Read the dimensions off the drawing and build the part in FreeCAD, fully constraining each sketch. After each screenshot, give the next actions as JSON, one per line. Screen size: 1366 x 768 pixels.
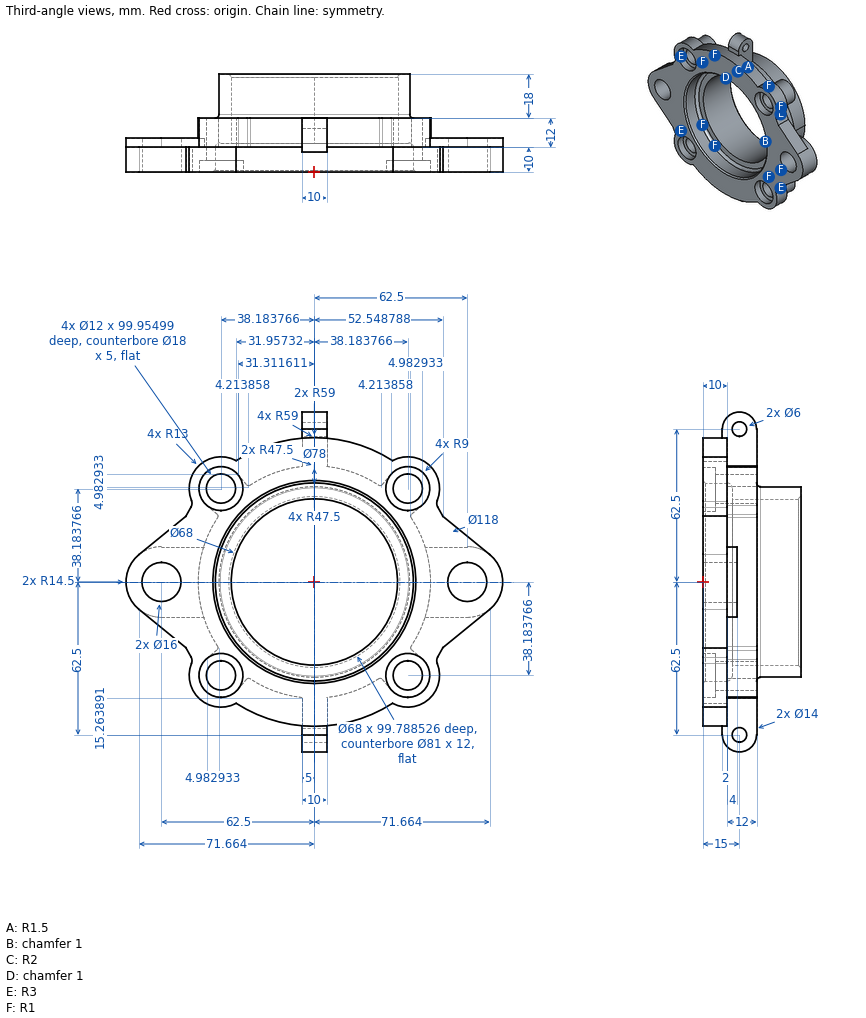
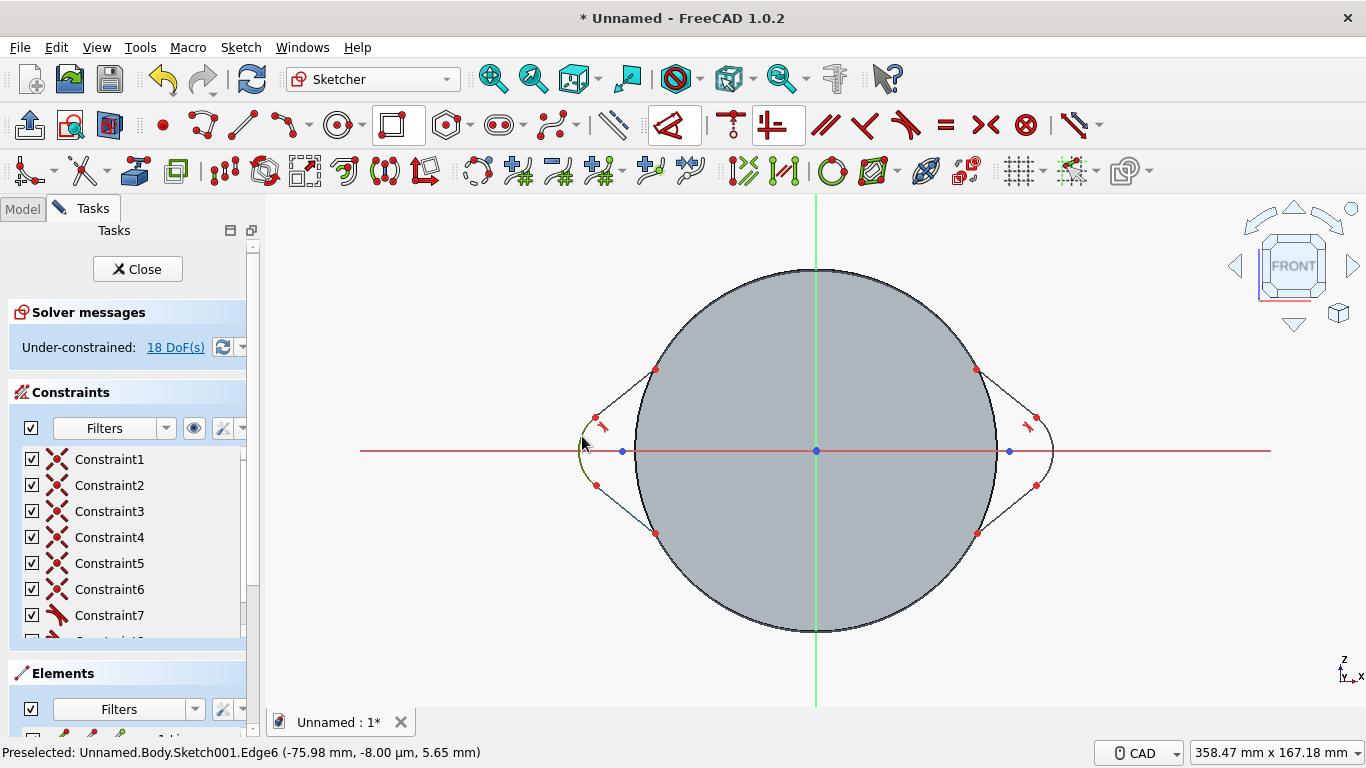
{"action": "left_click", "coordinate": [906, 126]}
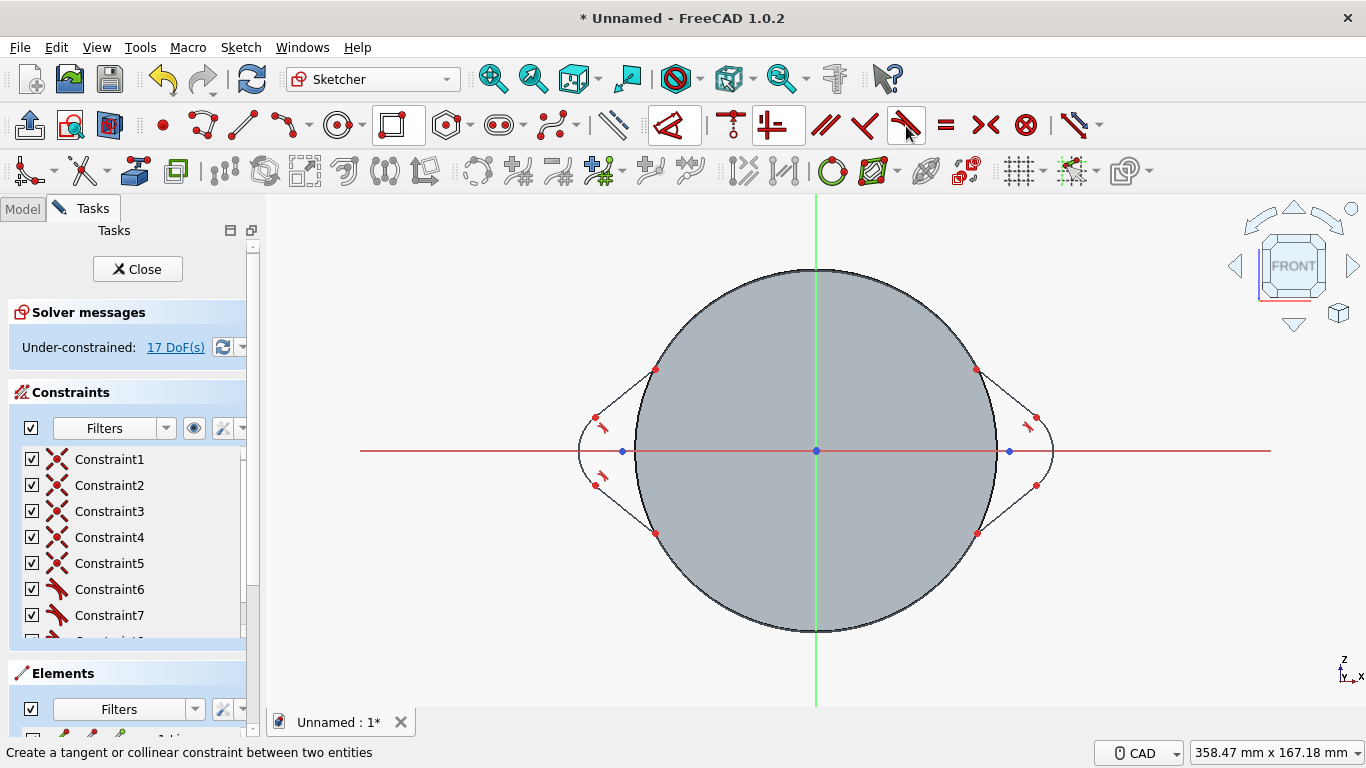
{"action": "left_click", "coordinate": [995, 520]}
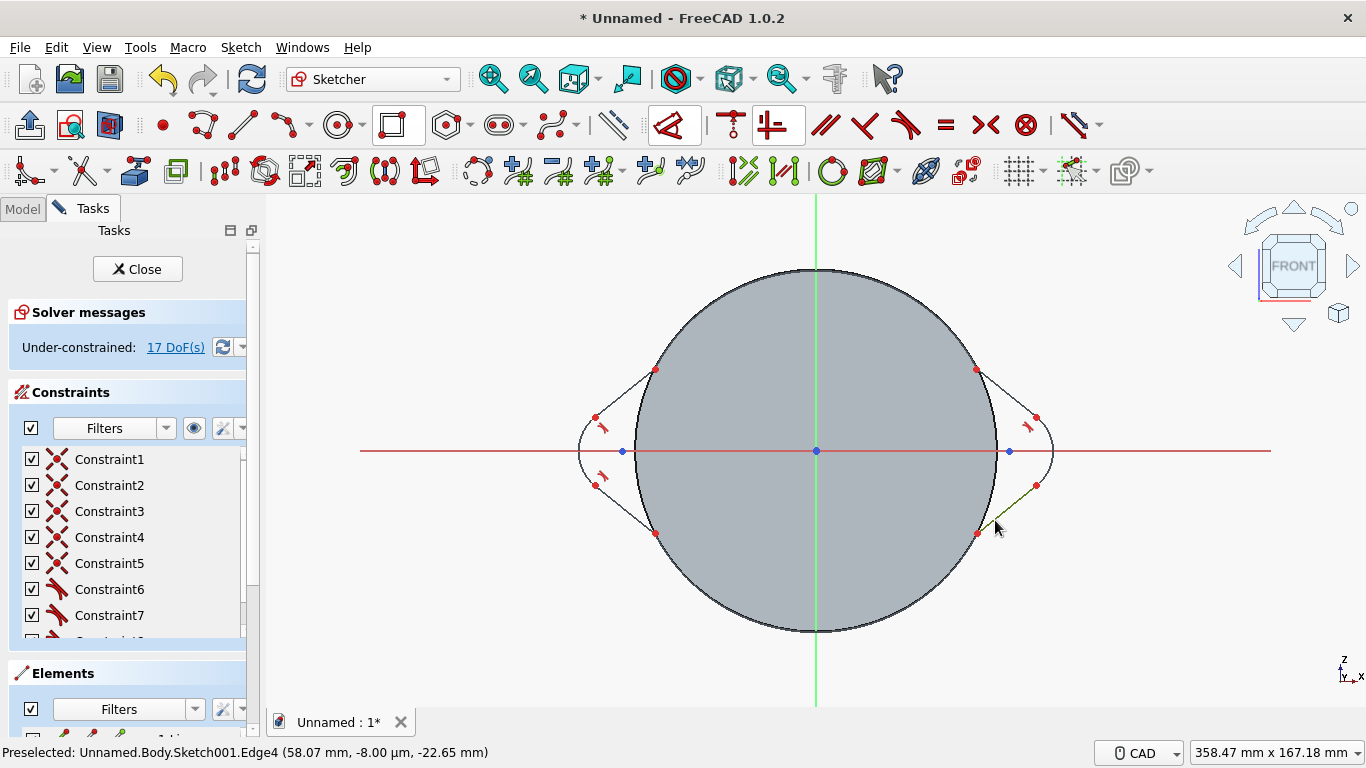
{"action": "left_click", "coordinate": [1050, 467]}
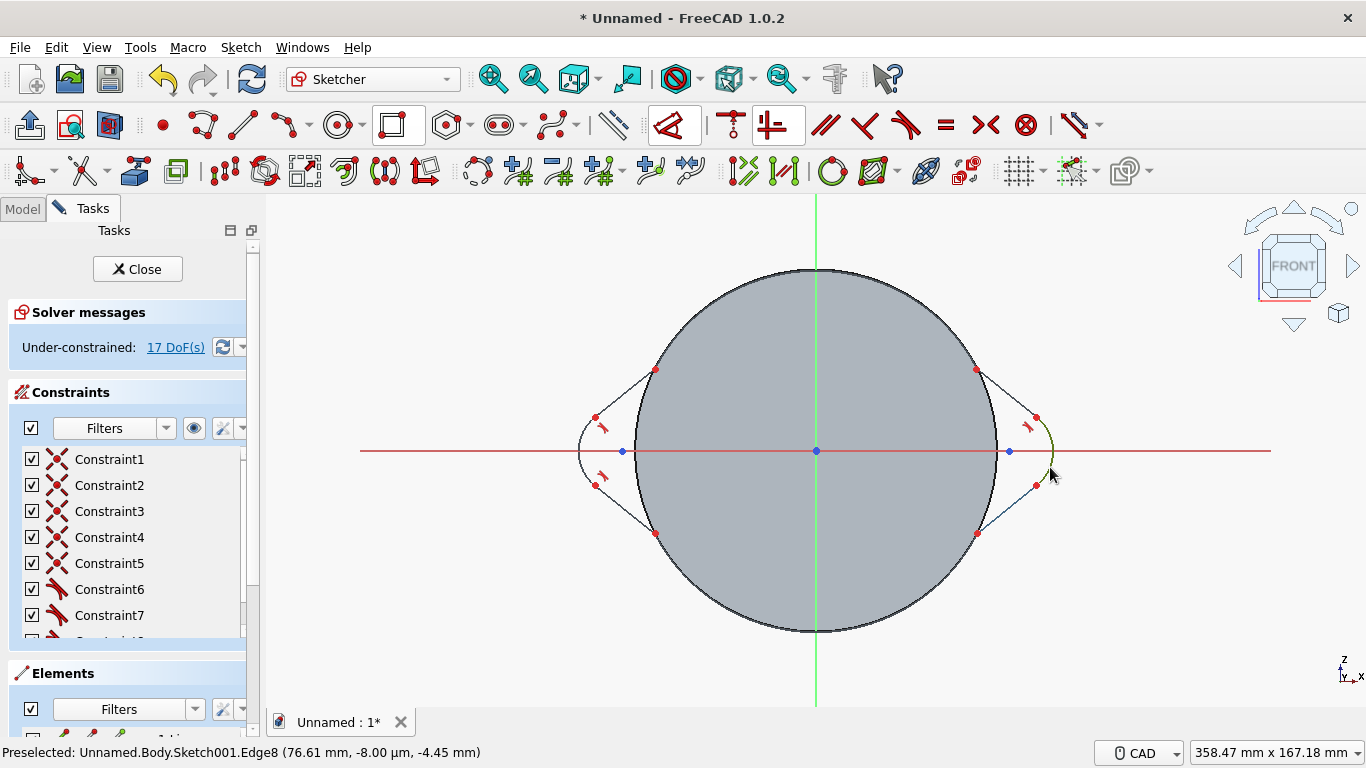
{"action": "left_click", "coordinate": [906, 126]}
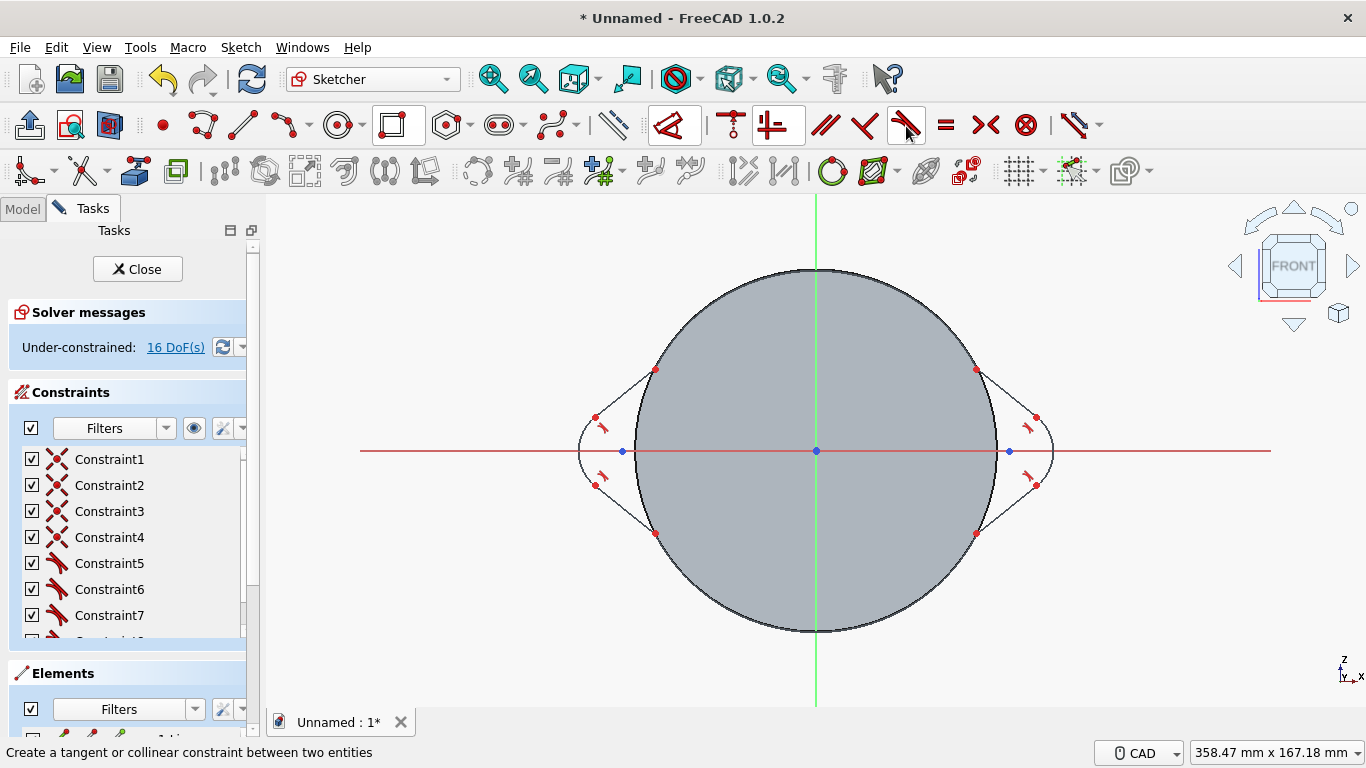
{"action": "left_click", "coordinate": [893, 288]}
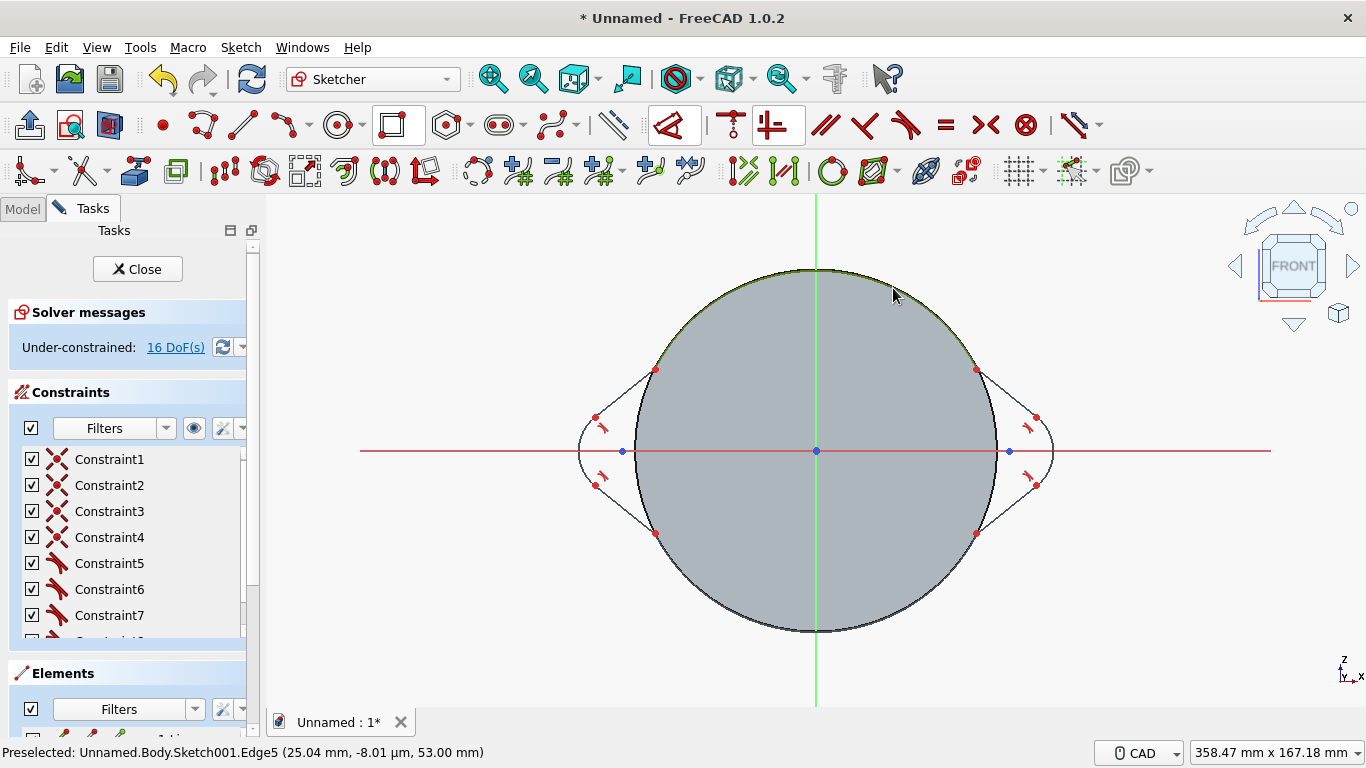
{"action": "left_click", "coordinate": [739, 615]}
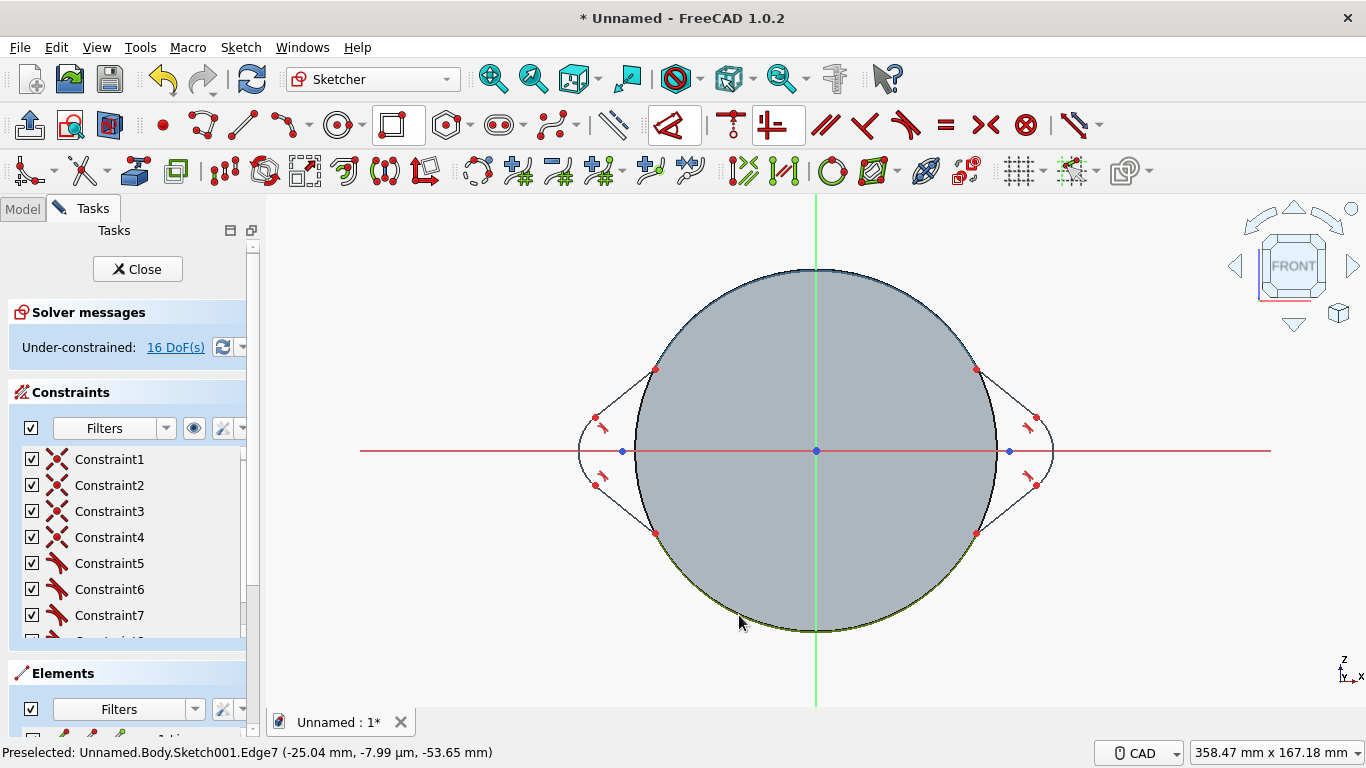
{"action": "left_click", "coordinate": [732, 126]}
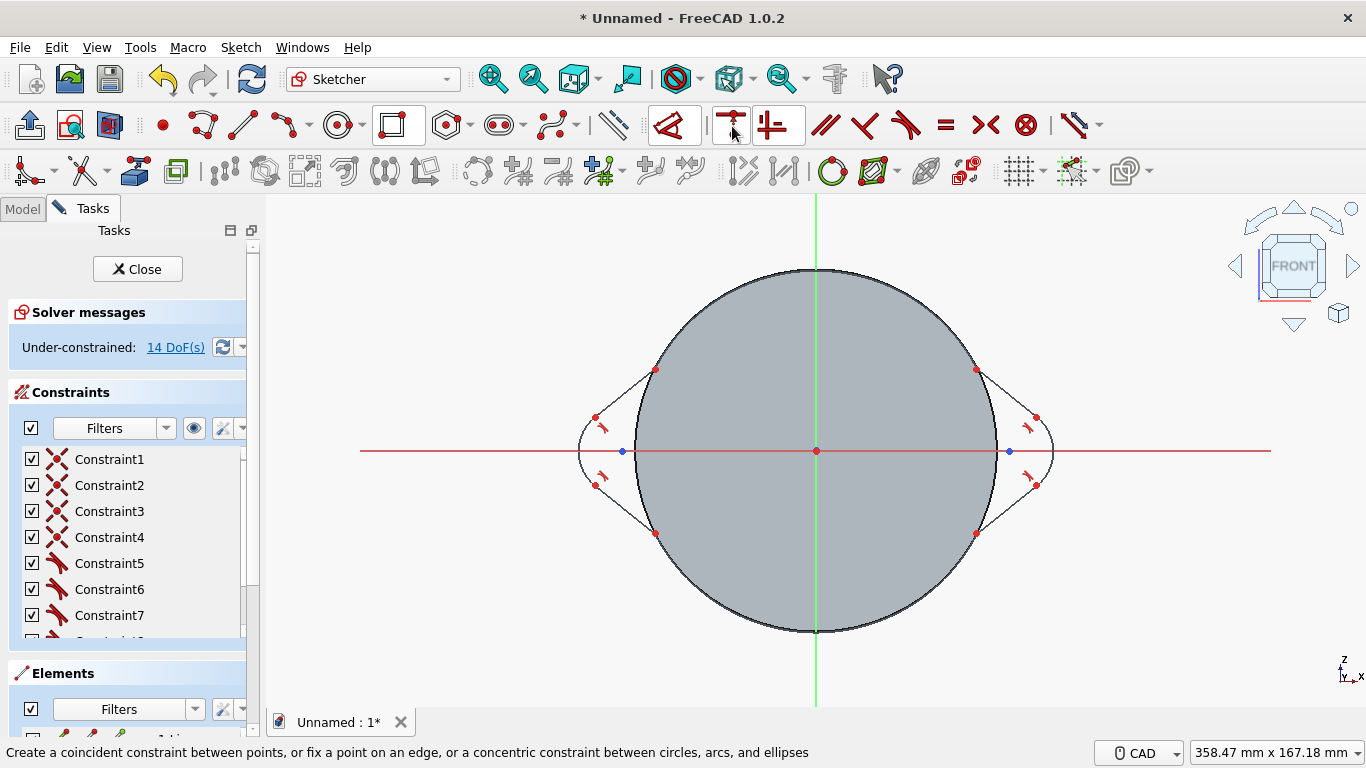
{"action": "left_click_drag", "start_coordinate": [806, 440], "coordinate": [826, 462]}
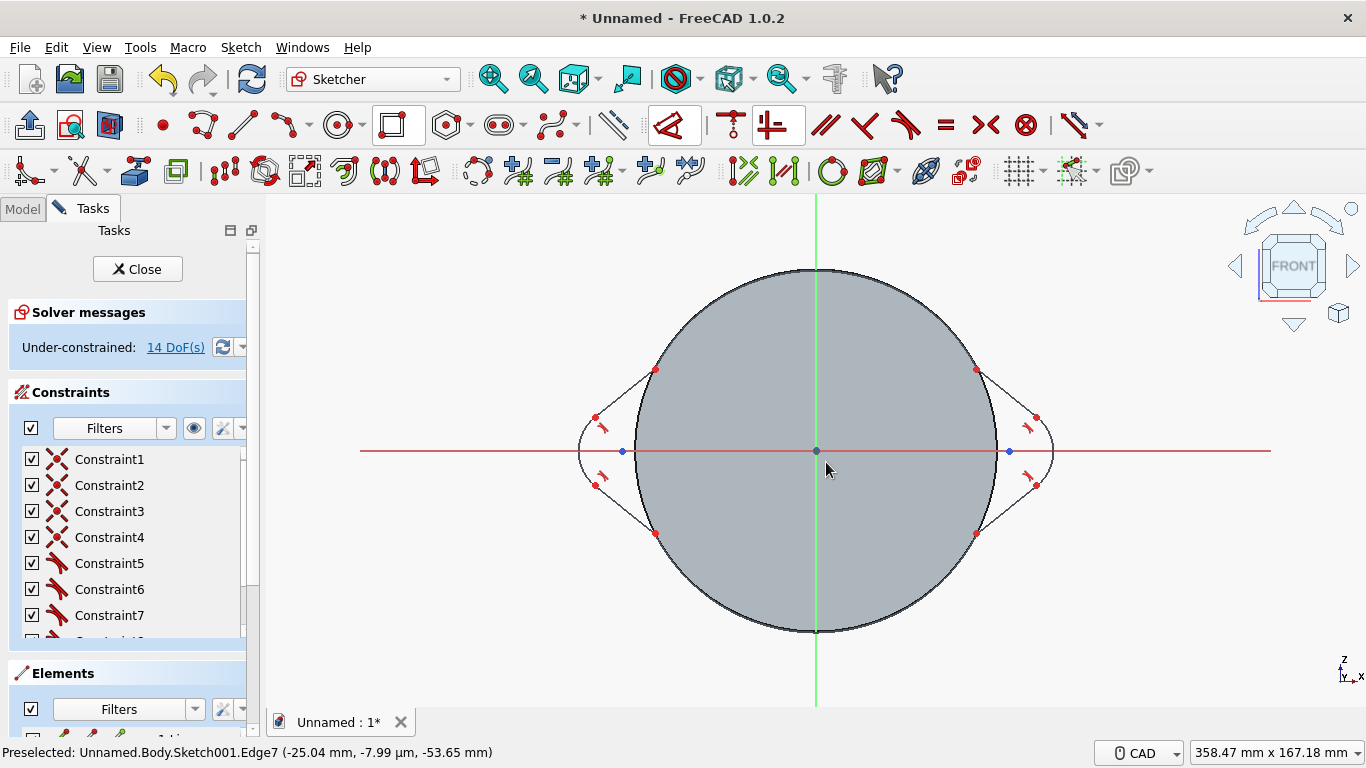
{"action": "left_click", "coordinate": [732, 126]}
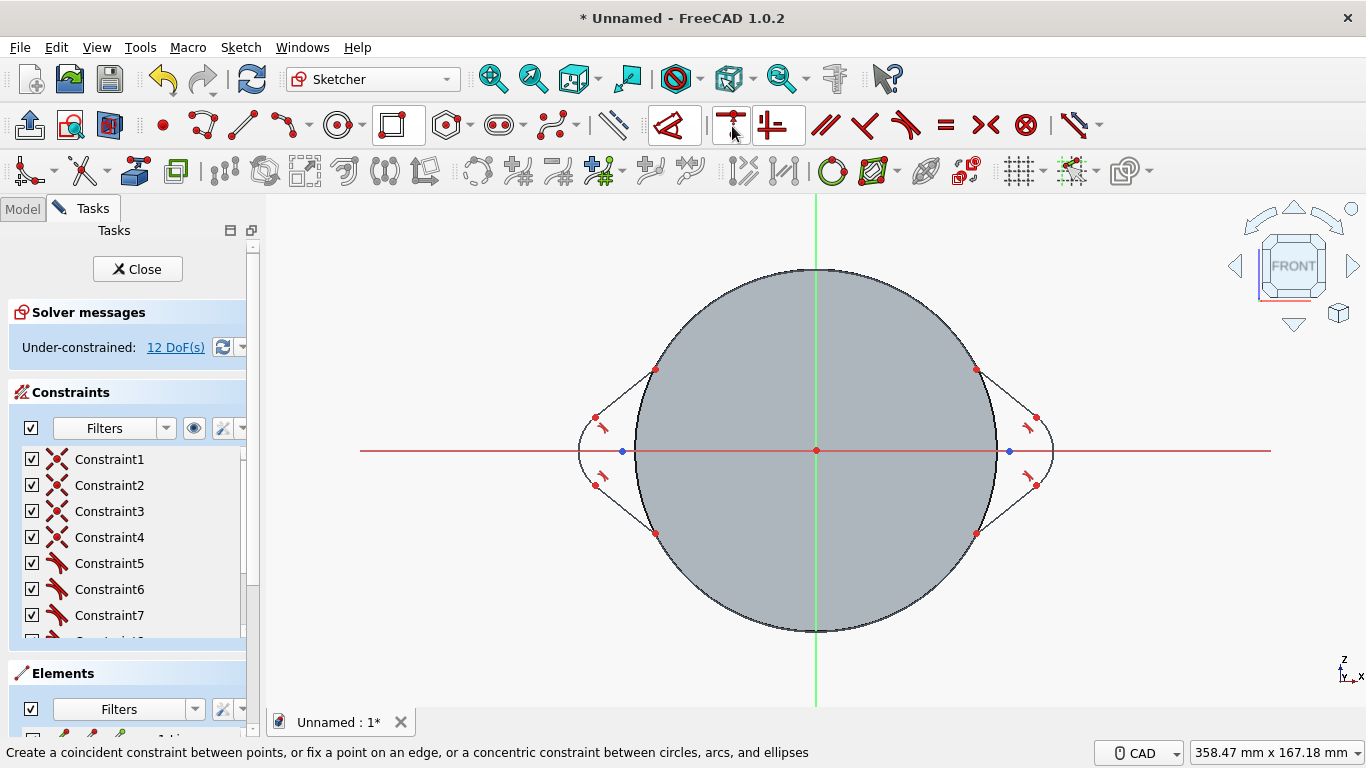
{"action": "left_click", "coordinate": [893, 287]}